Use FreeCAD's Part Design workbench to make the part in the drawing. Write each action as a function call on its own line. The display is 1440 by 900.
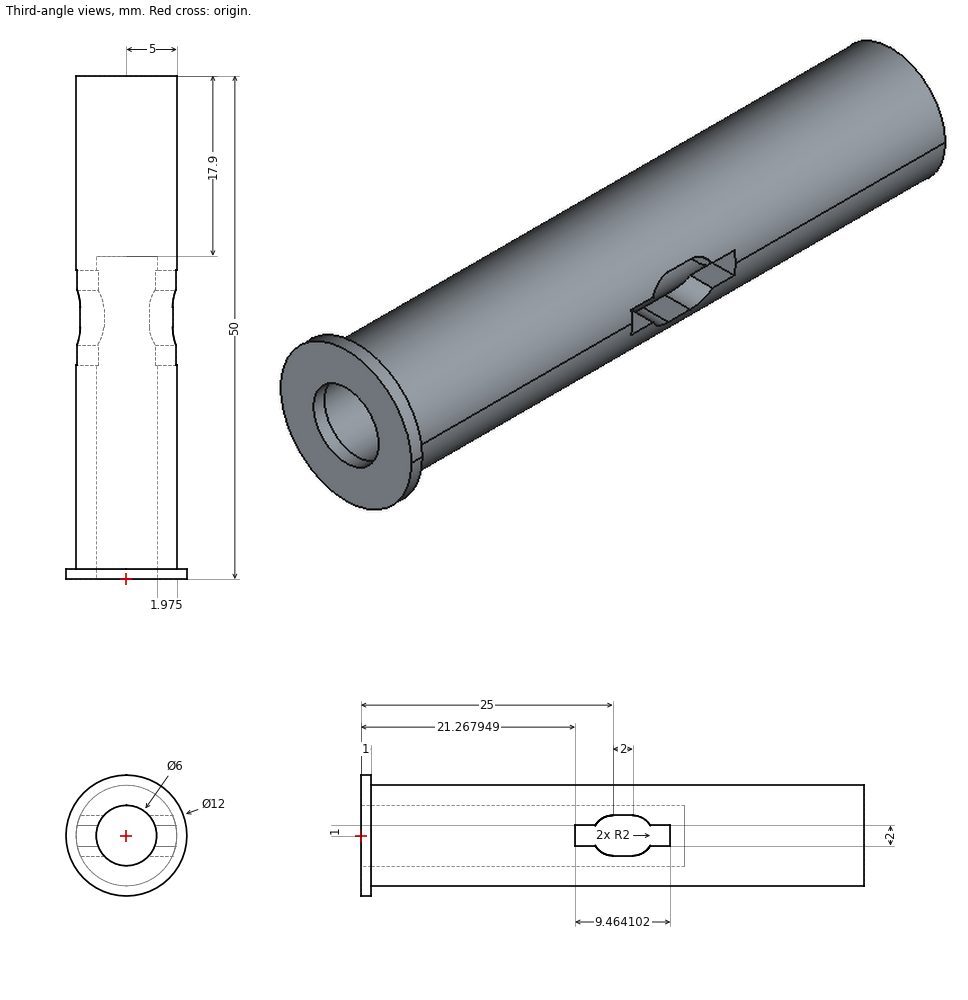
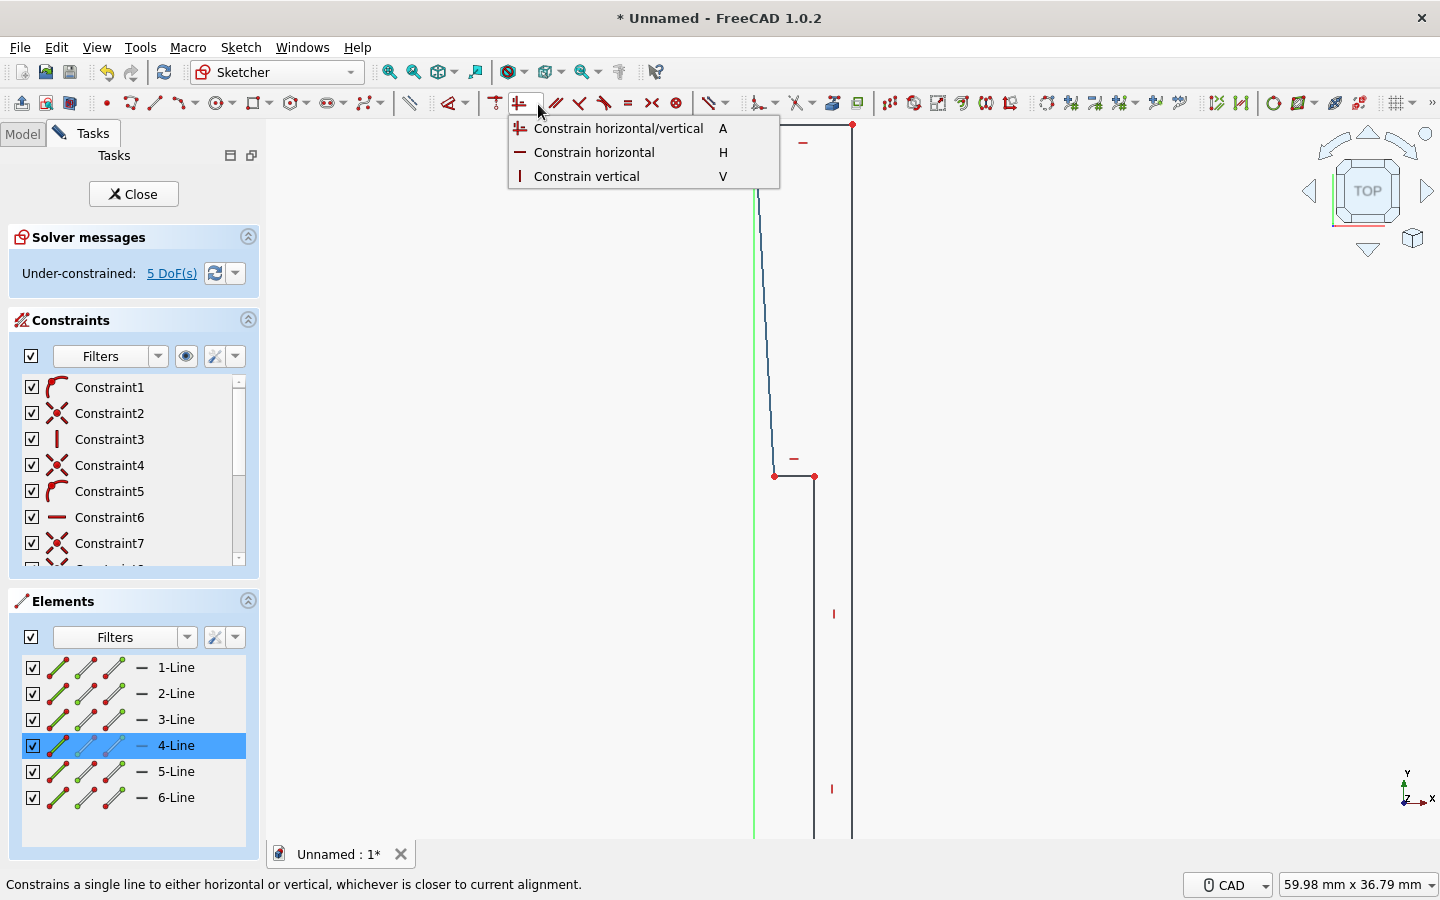
click(644, 176)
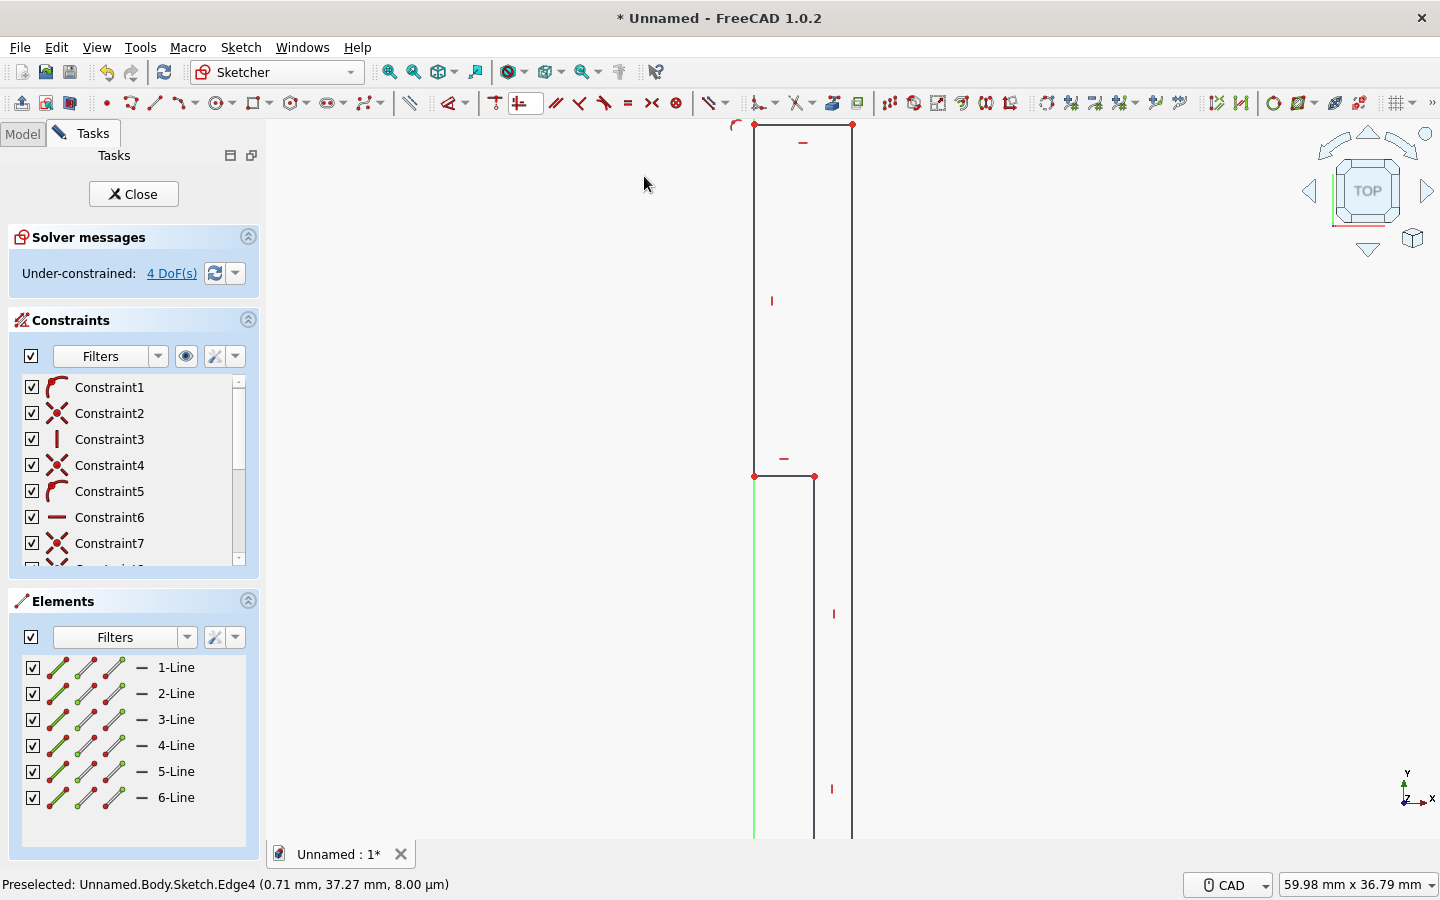
scroll(769, 370, down, 4)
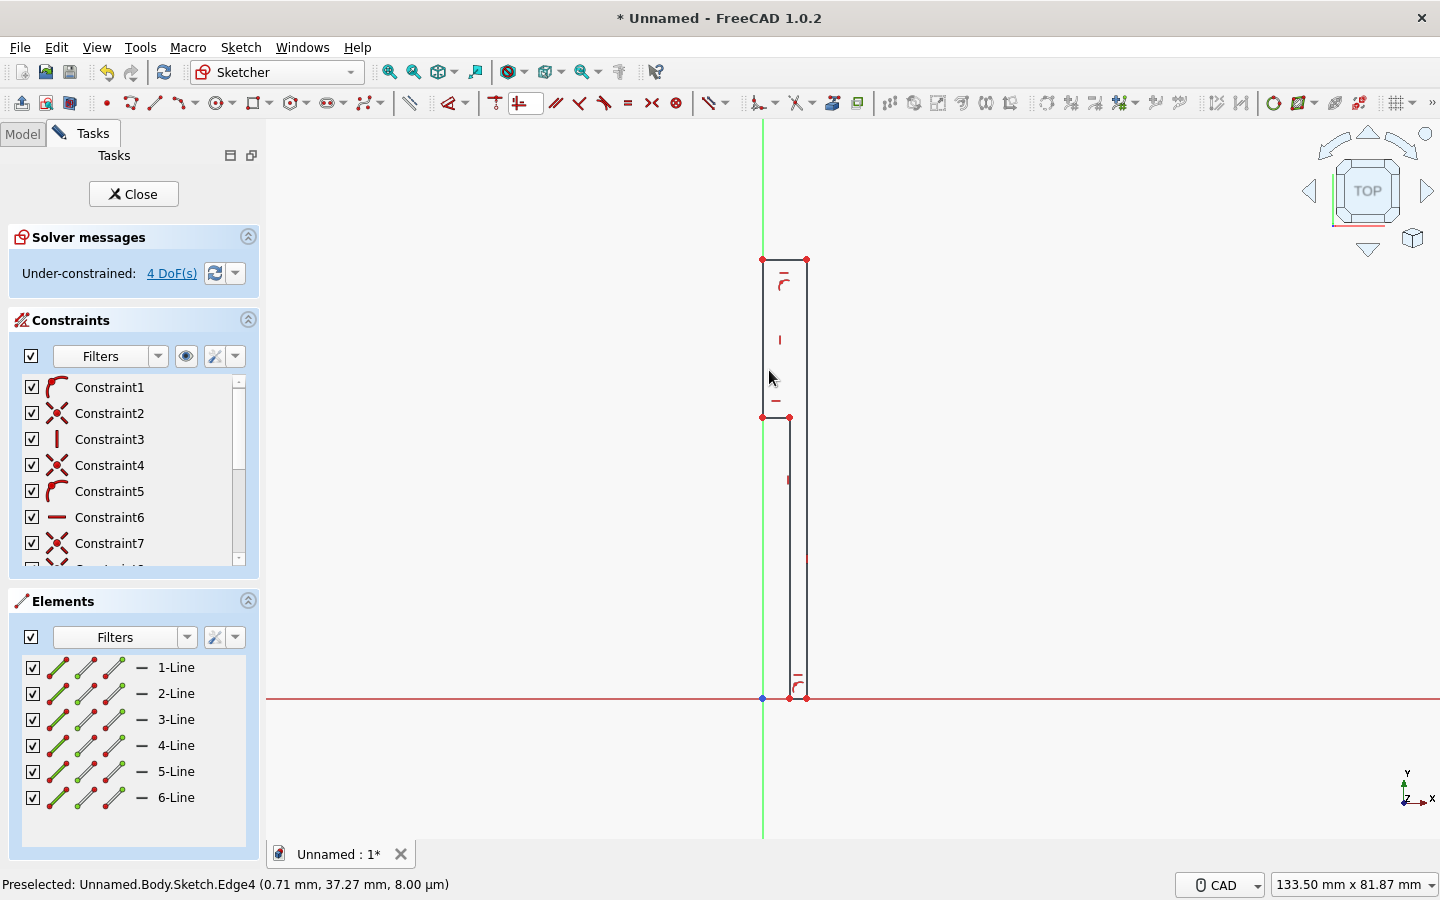
click(793, 260)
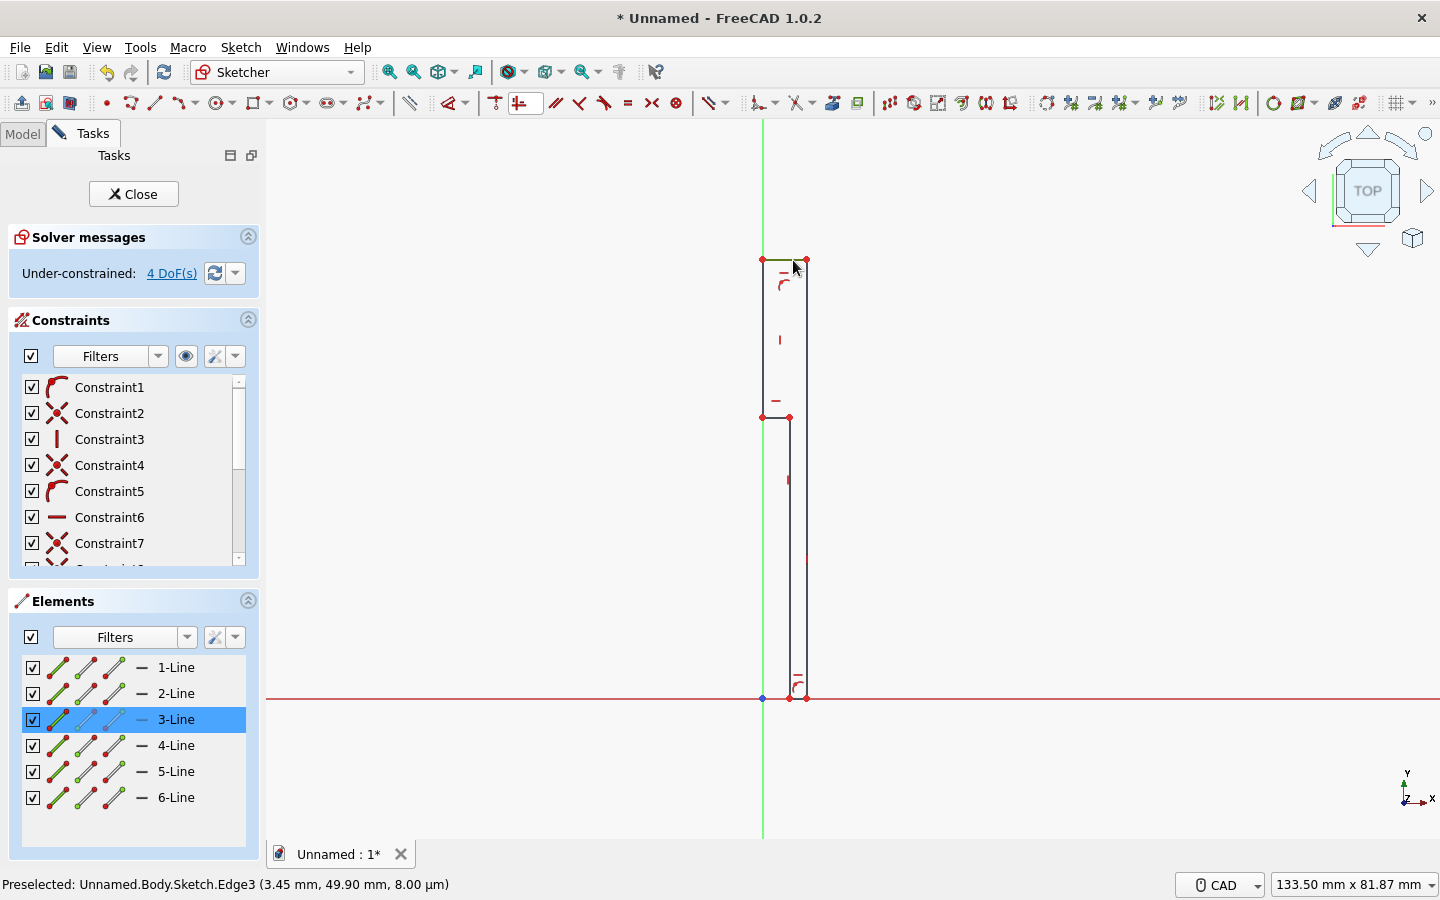
key(l)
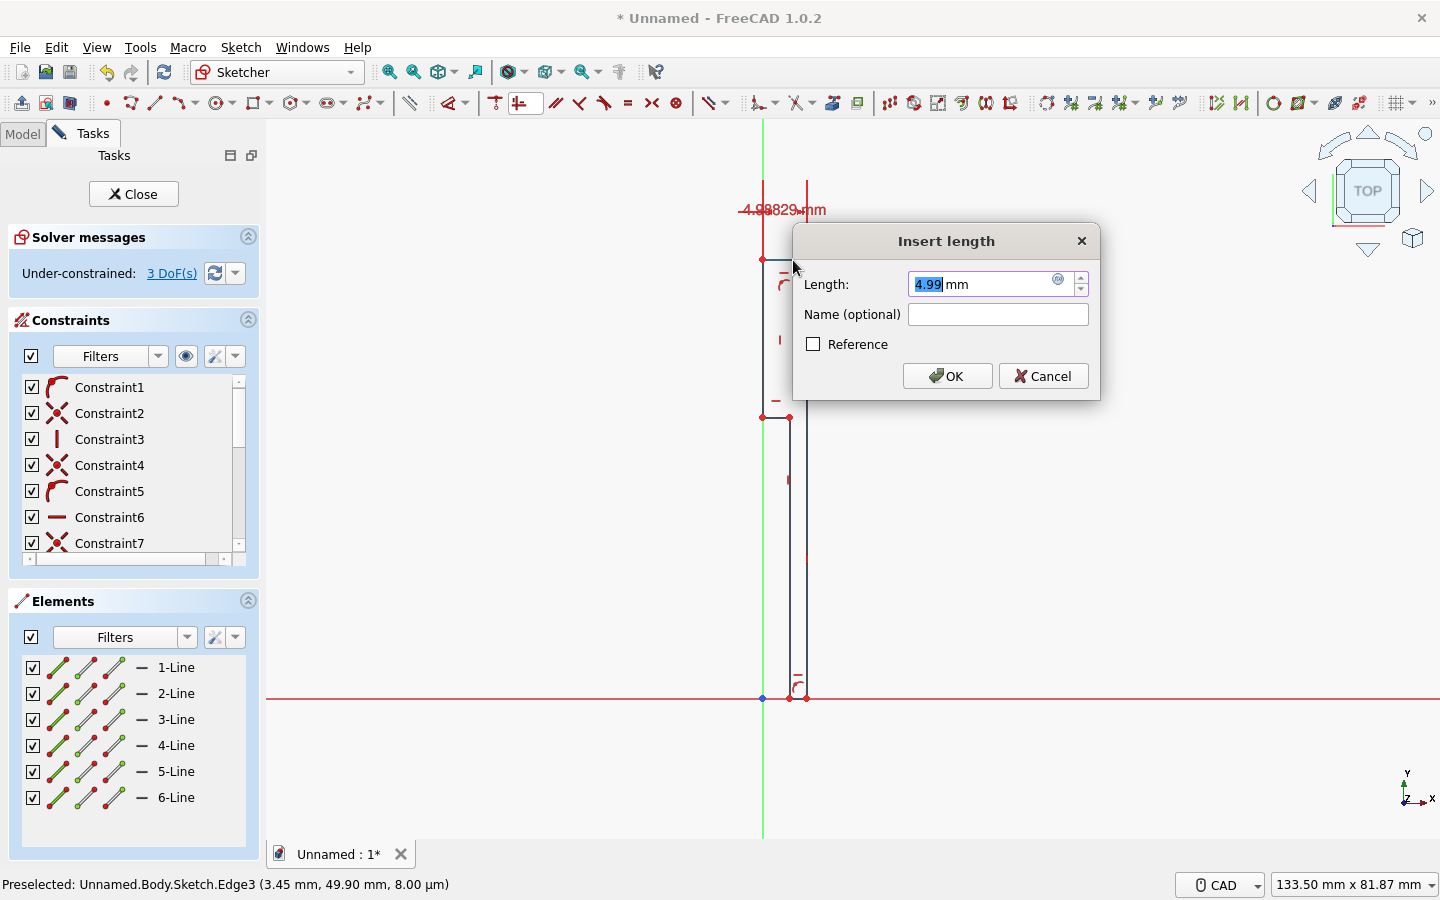
text(5)
key(Return)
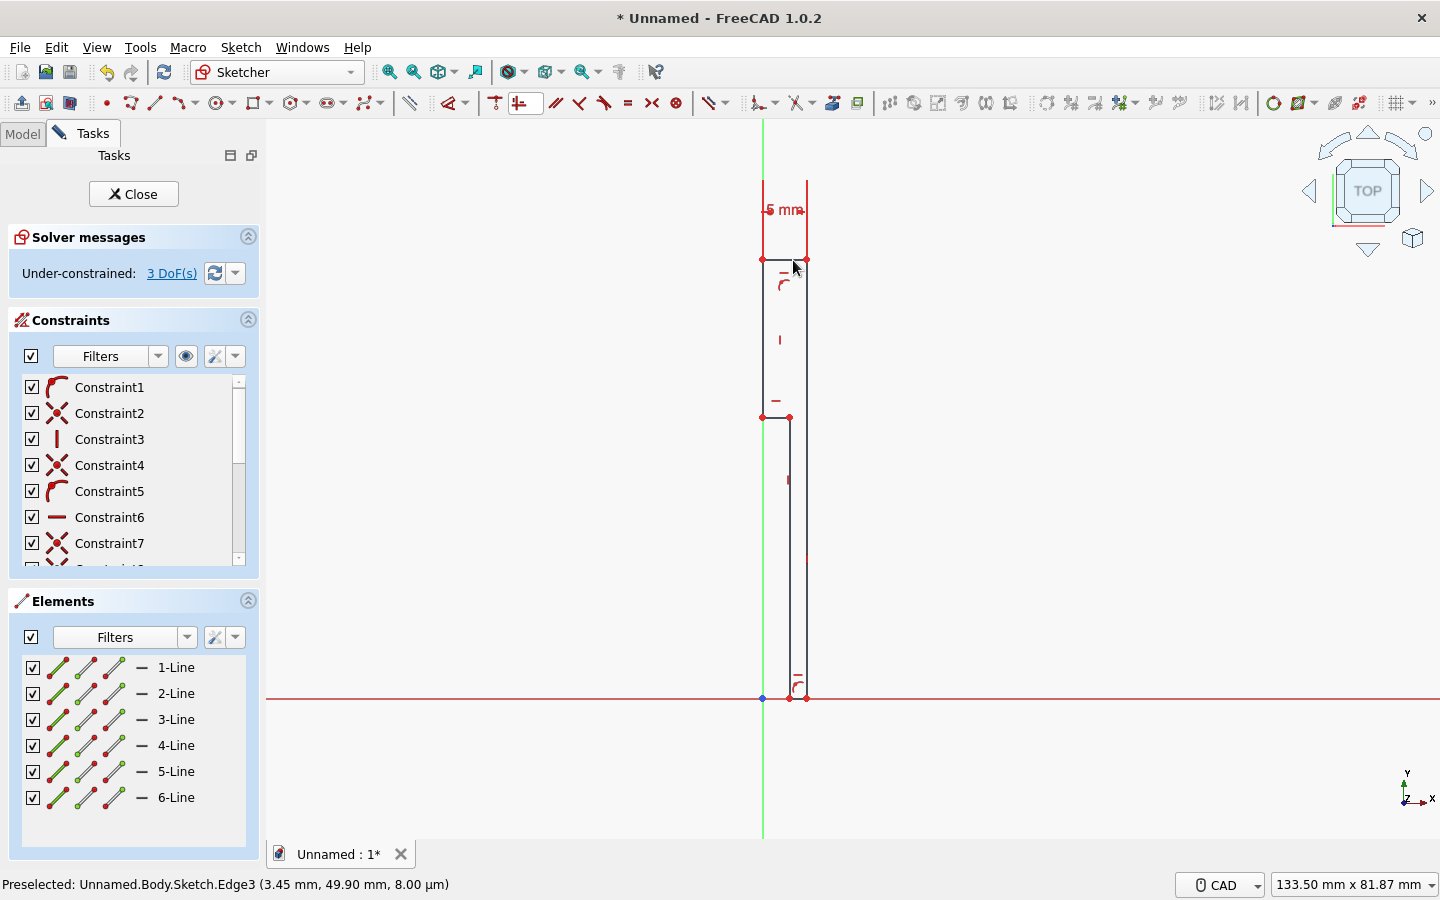
click(807, 567)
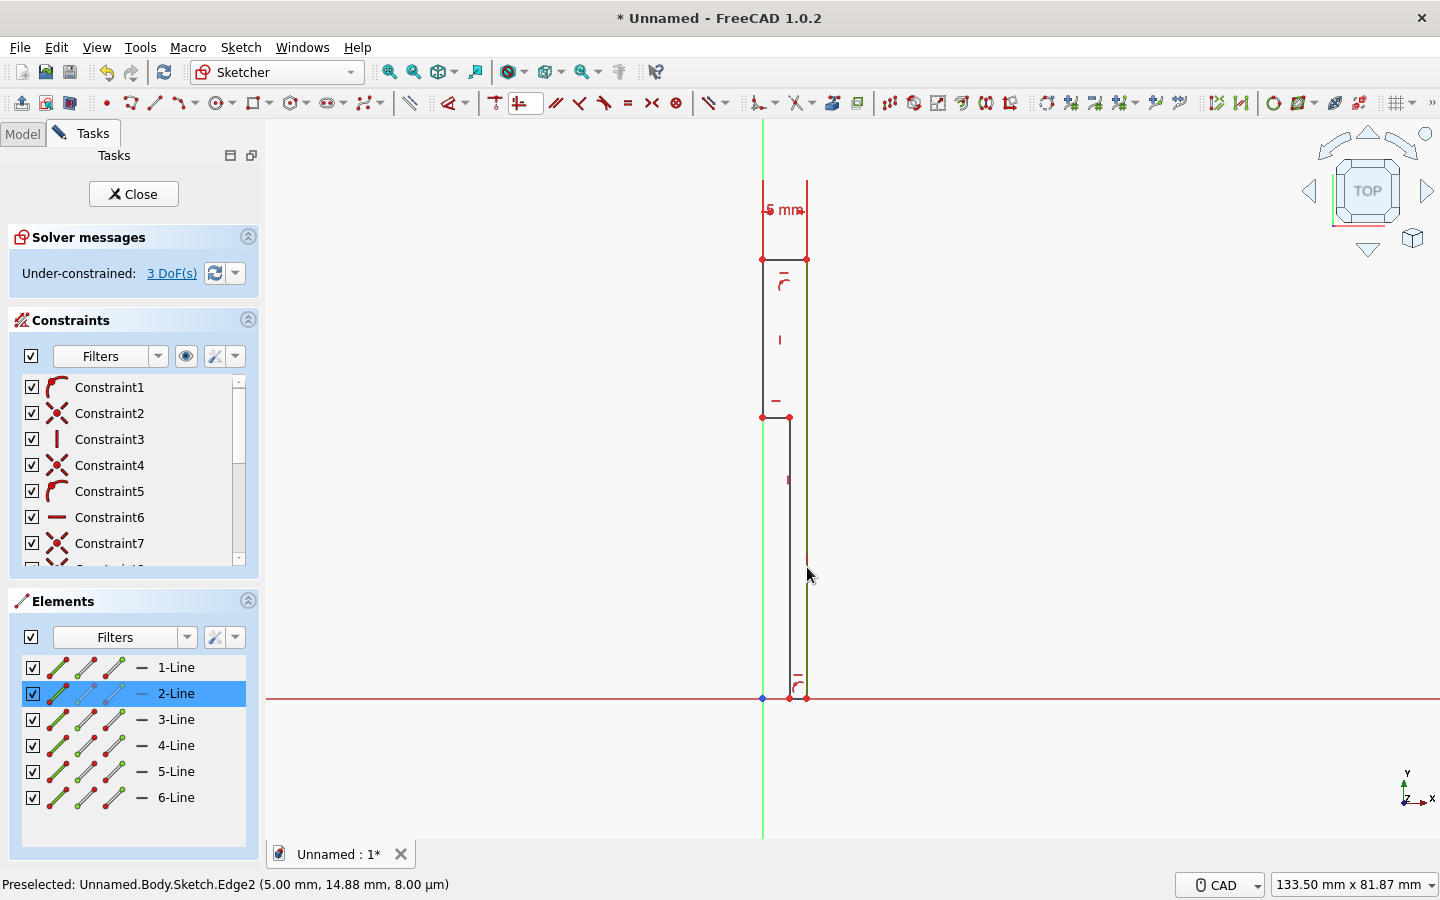
key(i)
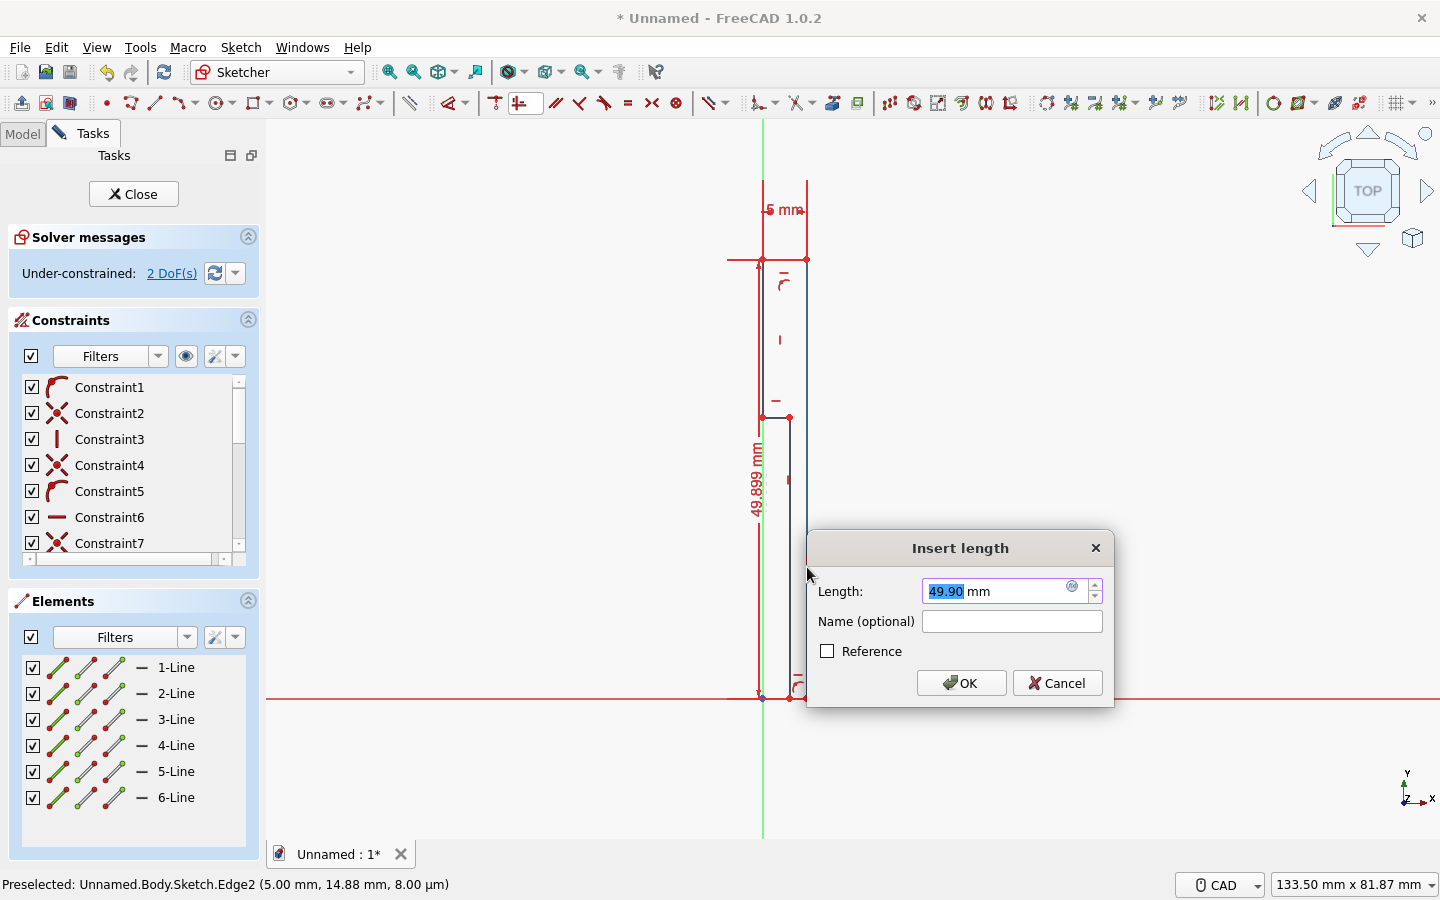
text(50)
key(Return)